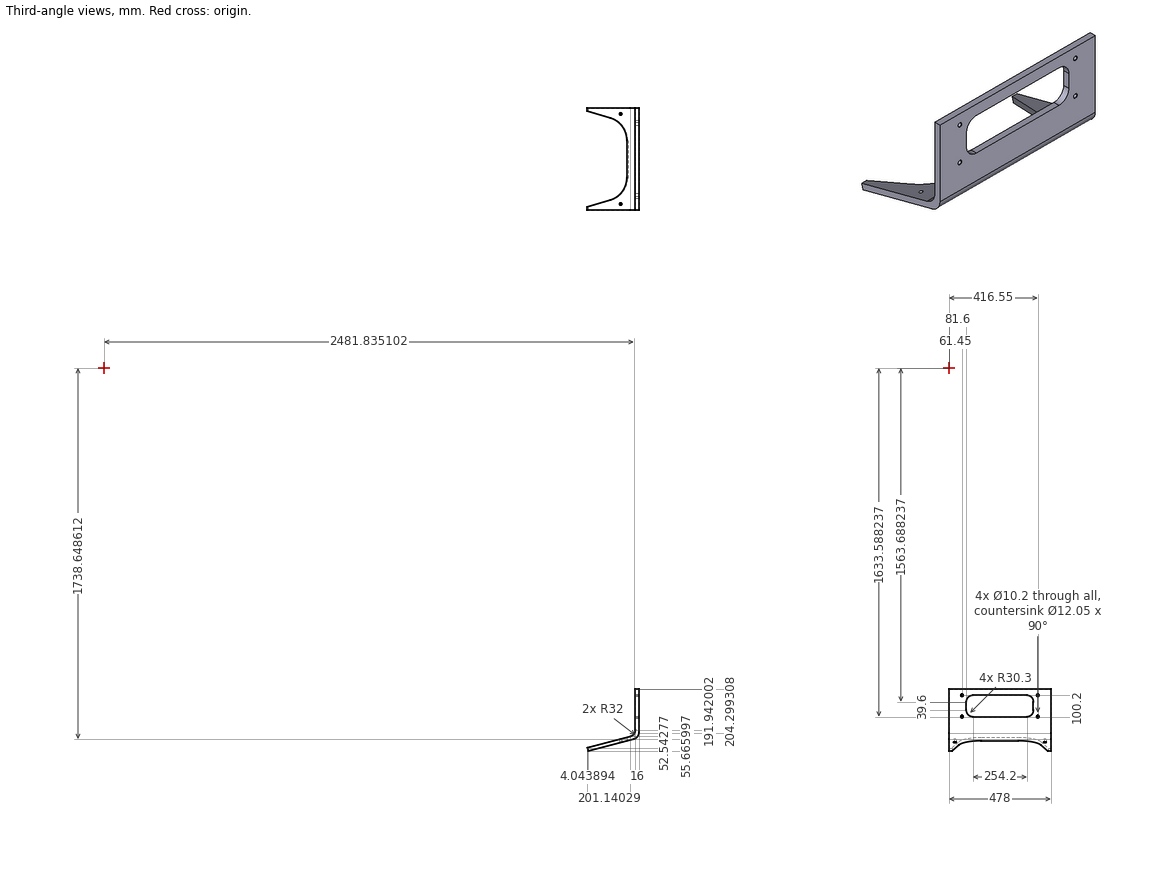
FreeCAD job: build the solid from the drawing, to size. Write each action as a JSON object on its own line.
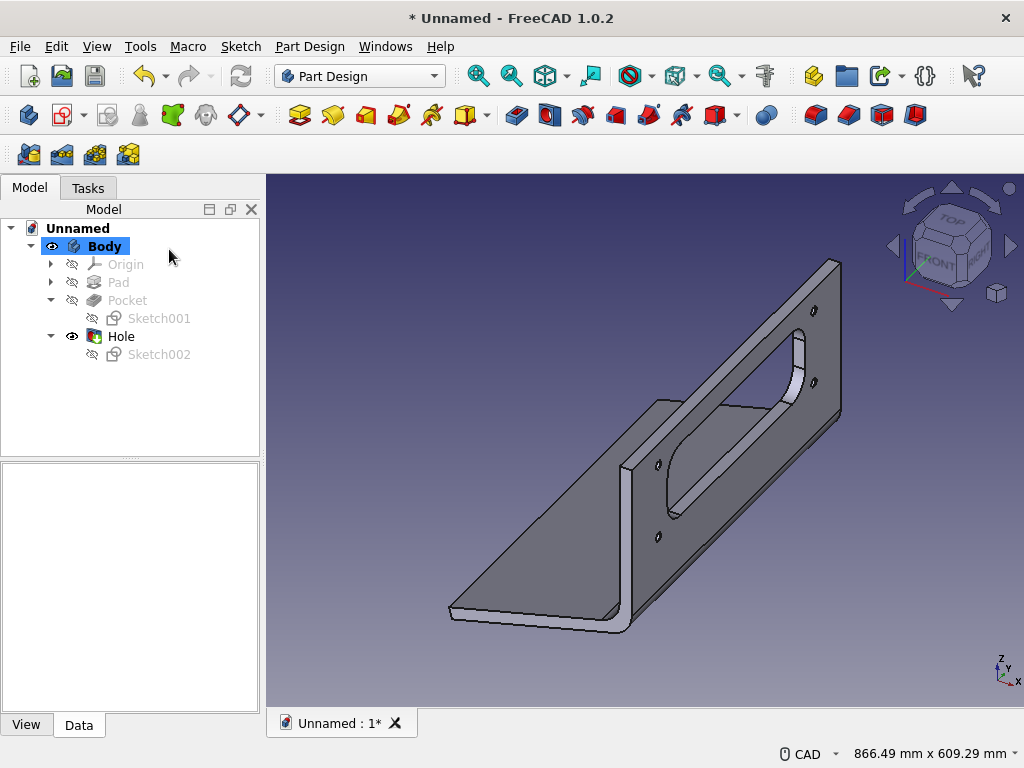
{"action": "key", "text": "5"}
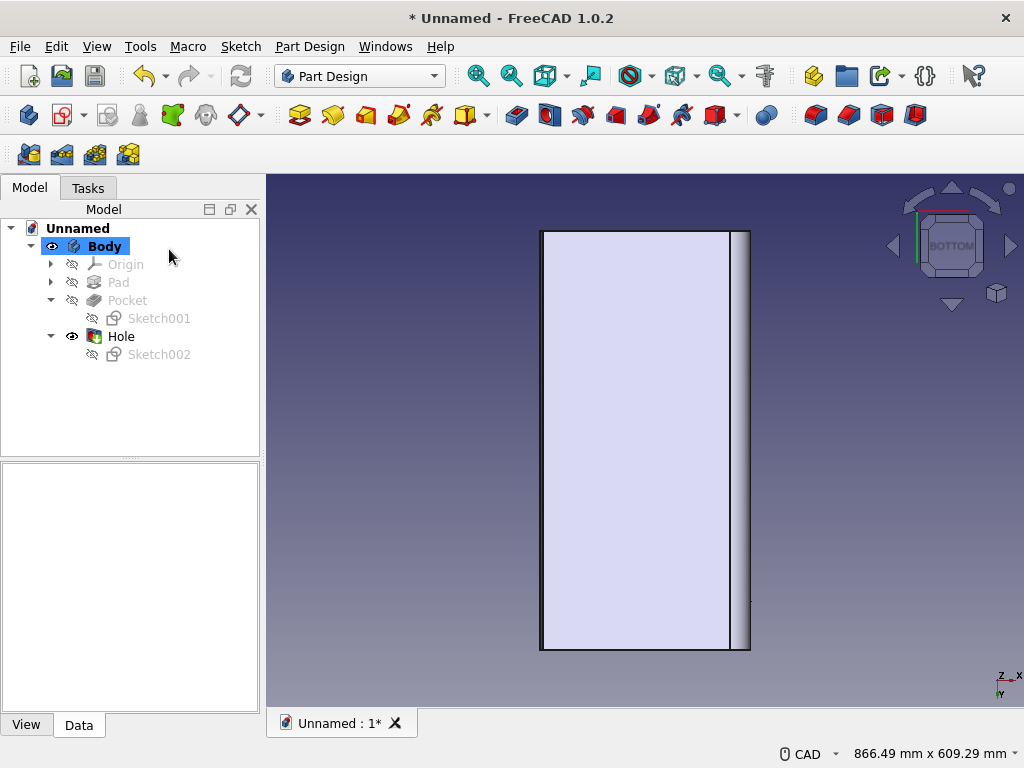
{"action": "left_click", "coordinate": [636, 439]}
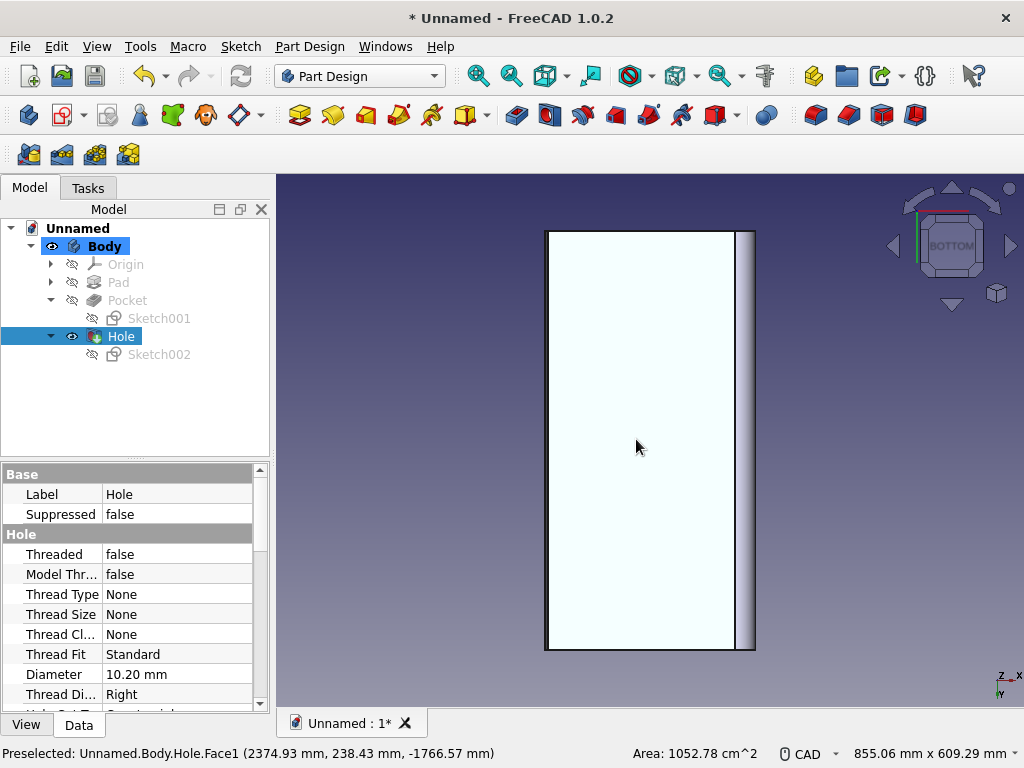
{"action": "left_click", "coordinate": [62, 116]}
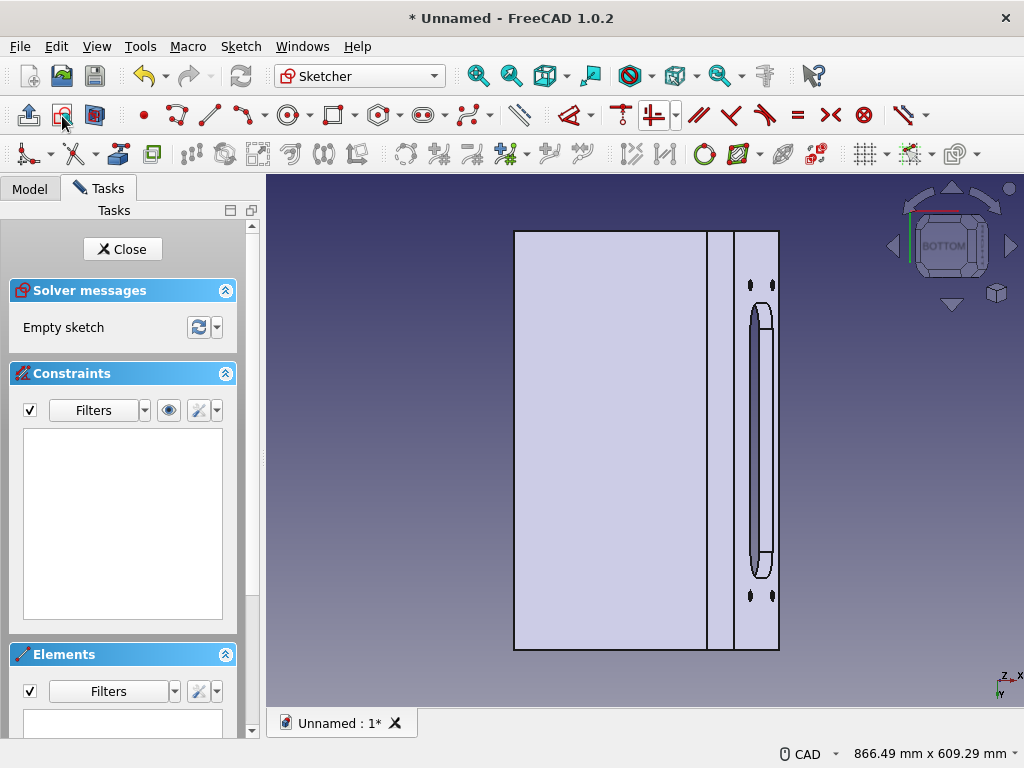
{"action": "left_click", "coordinate": [210, 116]}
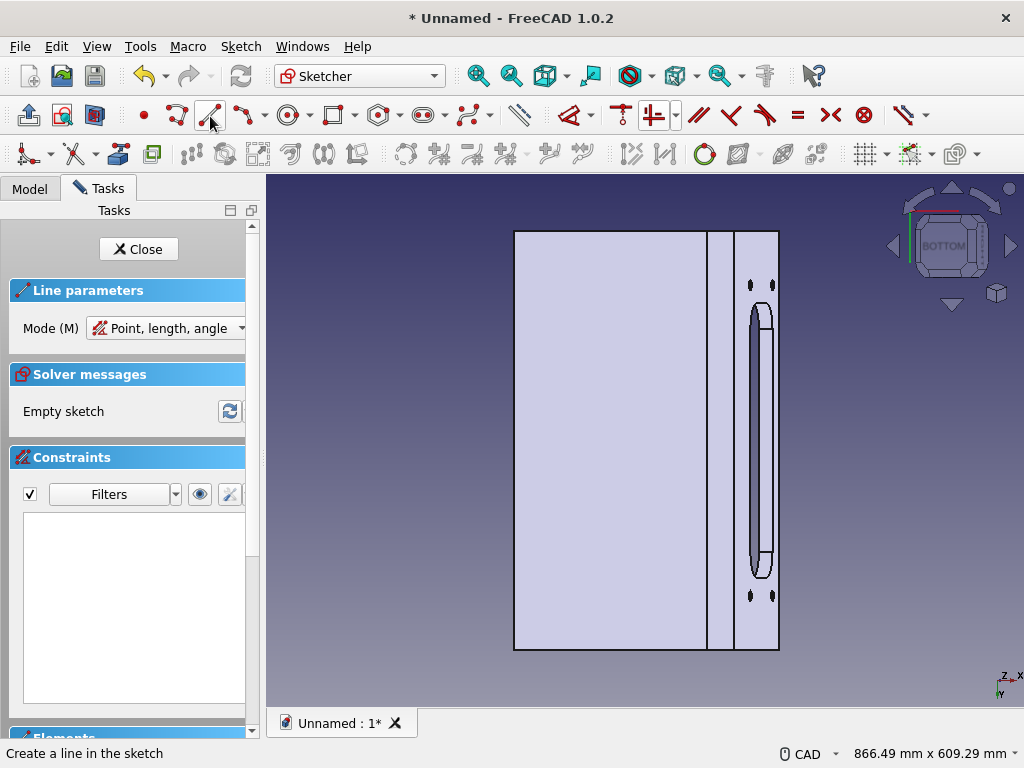
{"action": "left_click", "coordinate": [681, 517]}
{"action": "left_click", "coordinate": [681, 364]}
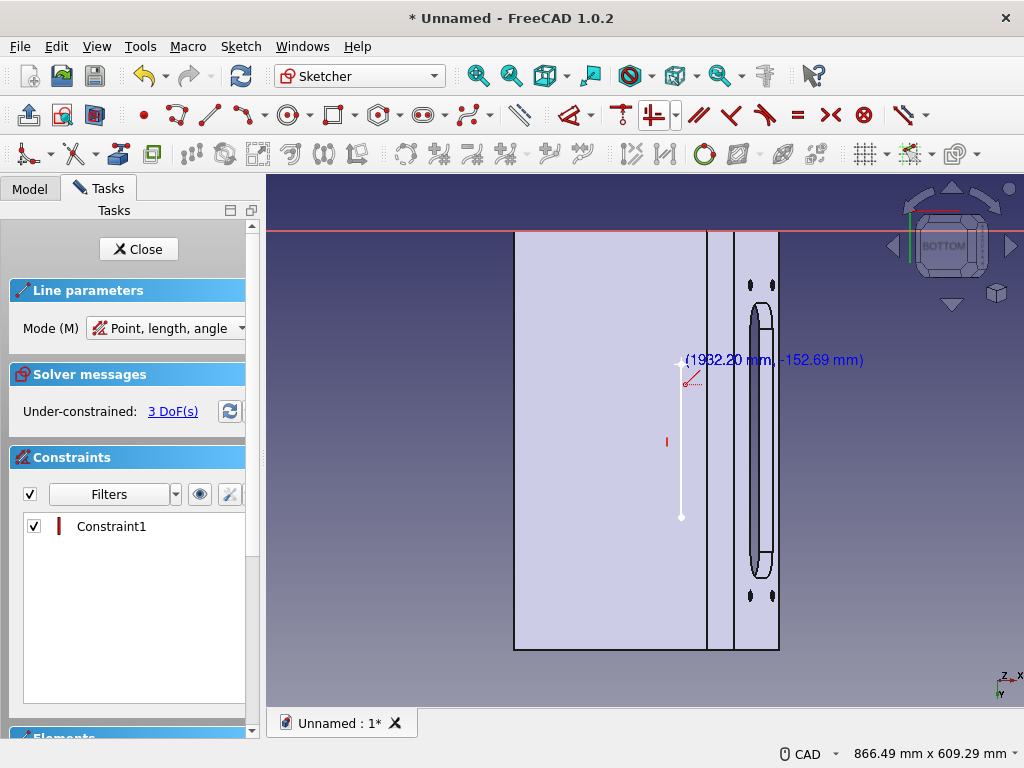
{"action": "left_click", "coordinate": [177, 116]}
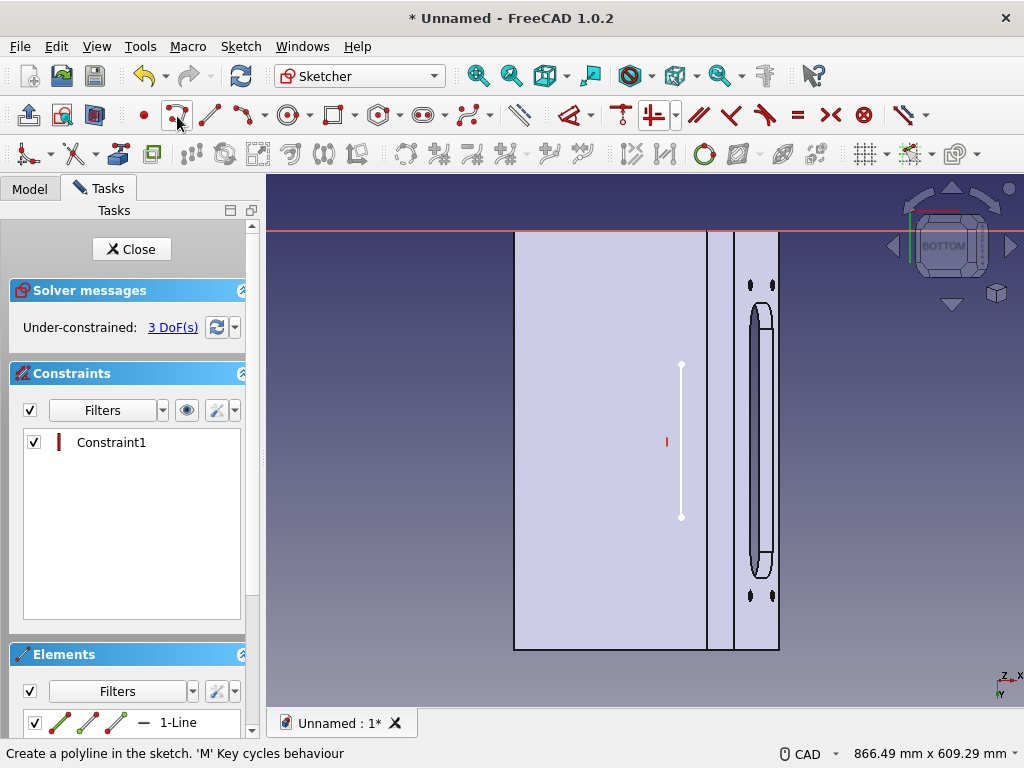
{"action": "left_click", "coordinate": [612, 273]}
{"action": "left_click", "coordinate": [514, 245]}
{"action": "left_click", "coordinate": [514, 636]}
{"action": "left_click", "coordinate": [612, 608]}
{"action": "right_click", "coordinate": [612, 608]}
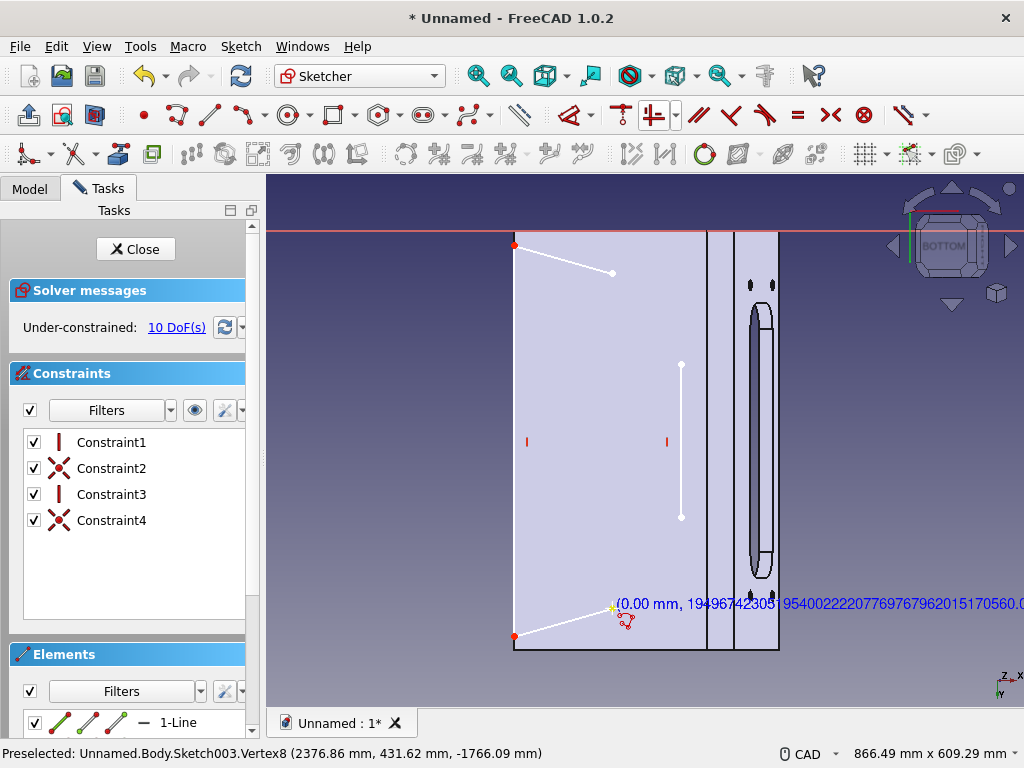
{"action": "left_click", "coordinate": [242, 116]}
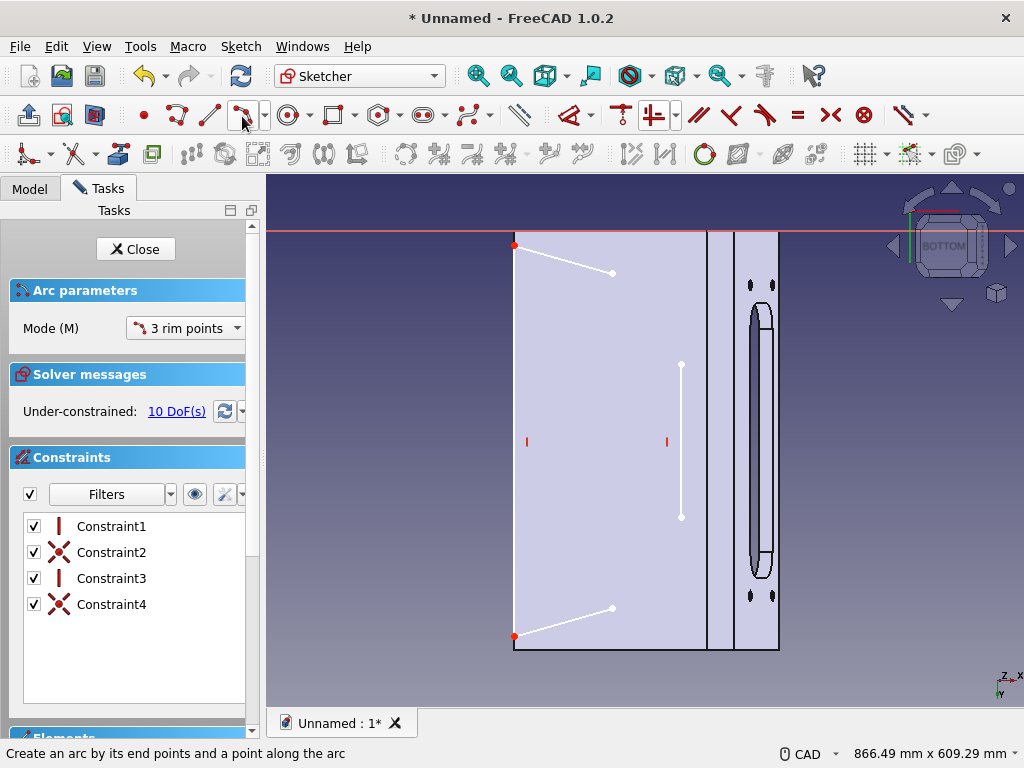
{"action": "left_click", "coordinate": [681, 365]}
{"action": "left_click", "coordinate": [612, 274]}
{"action": "left_click", "coordinate": [662, 307]}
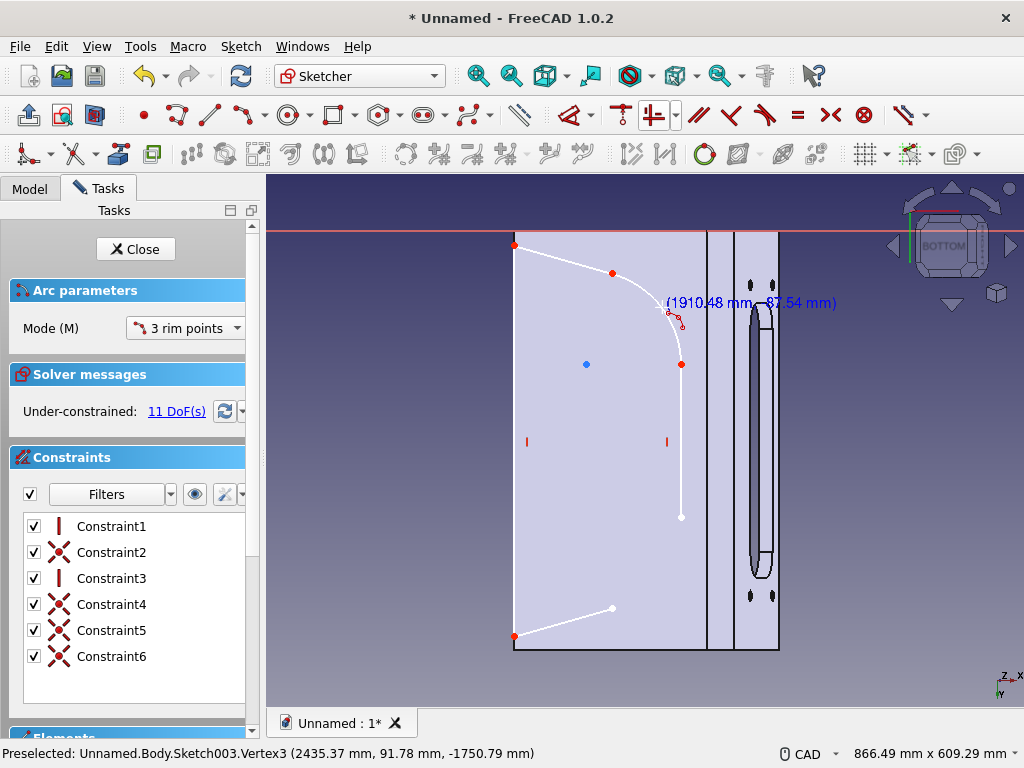
{"action": "left_click", "coordinate": [612, 609]}
{"action": "left_click", "coordinate": [681, 518]}
{"action": "left_click", "coordinate": [662, 574]}
{"action": "key", "text": "Escape"}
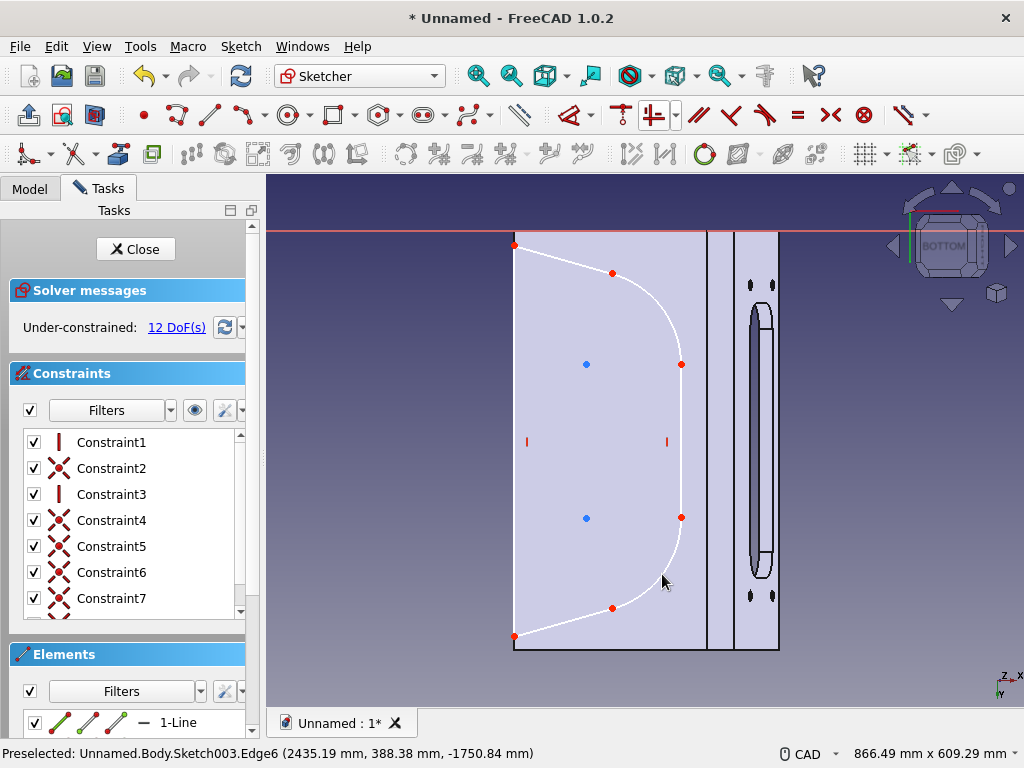
{"action": "left_click", "coordinate": [674, 329]}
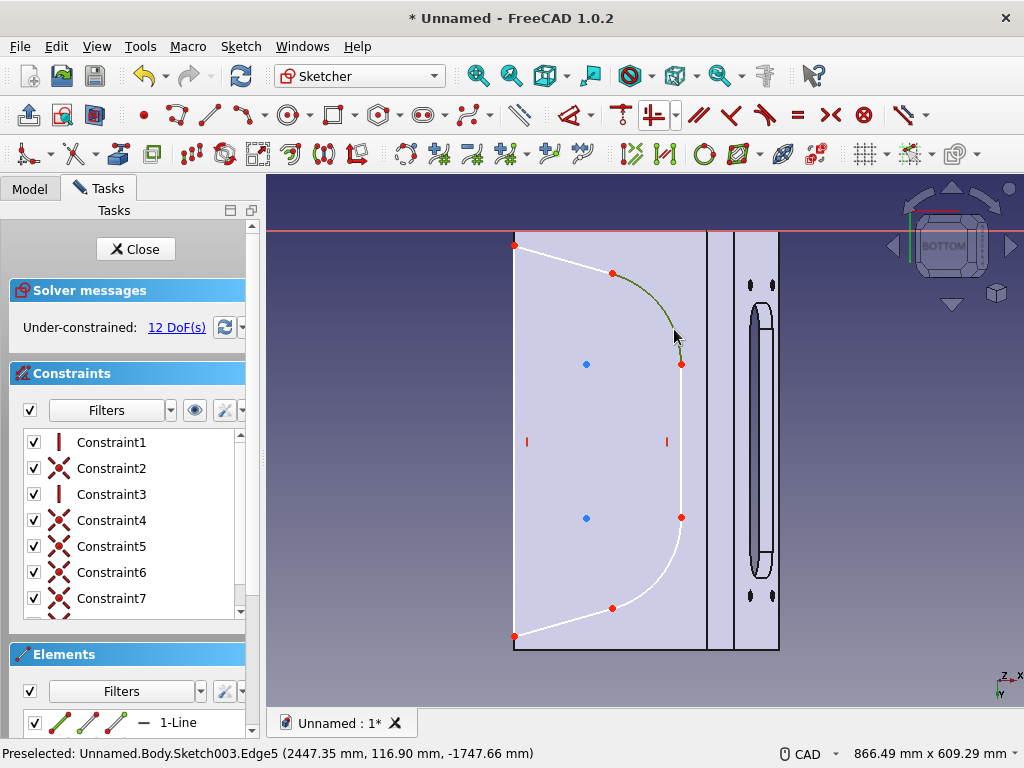
{"action": "left_click", "coordinate": [645, 593]}